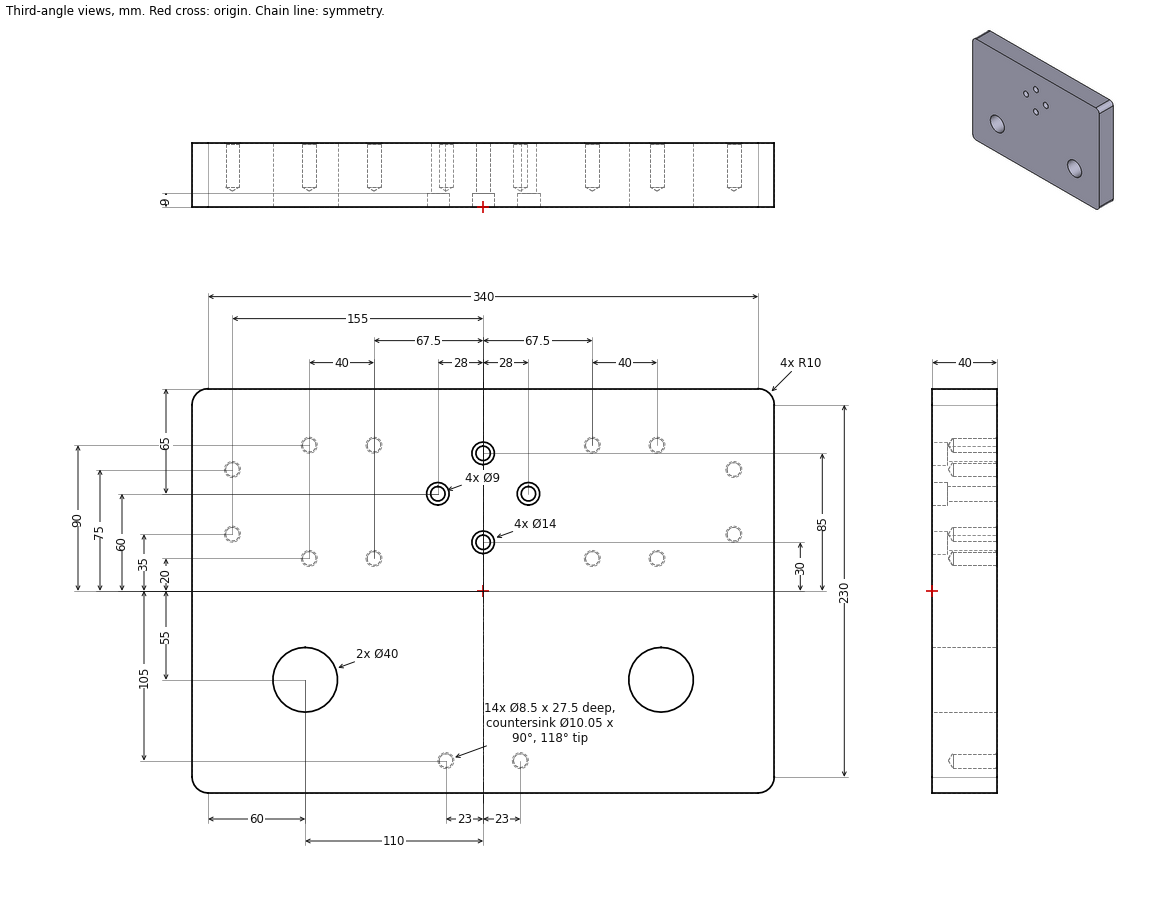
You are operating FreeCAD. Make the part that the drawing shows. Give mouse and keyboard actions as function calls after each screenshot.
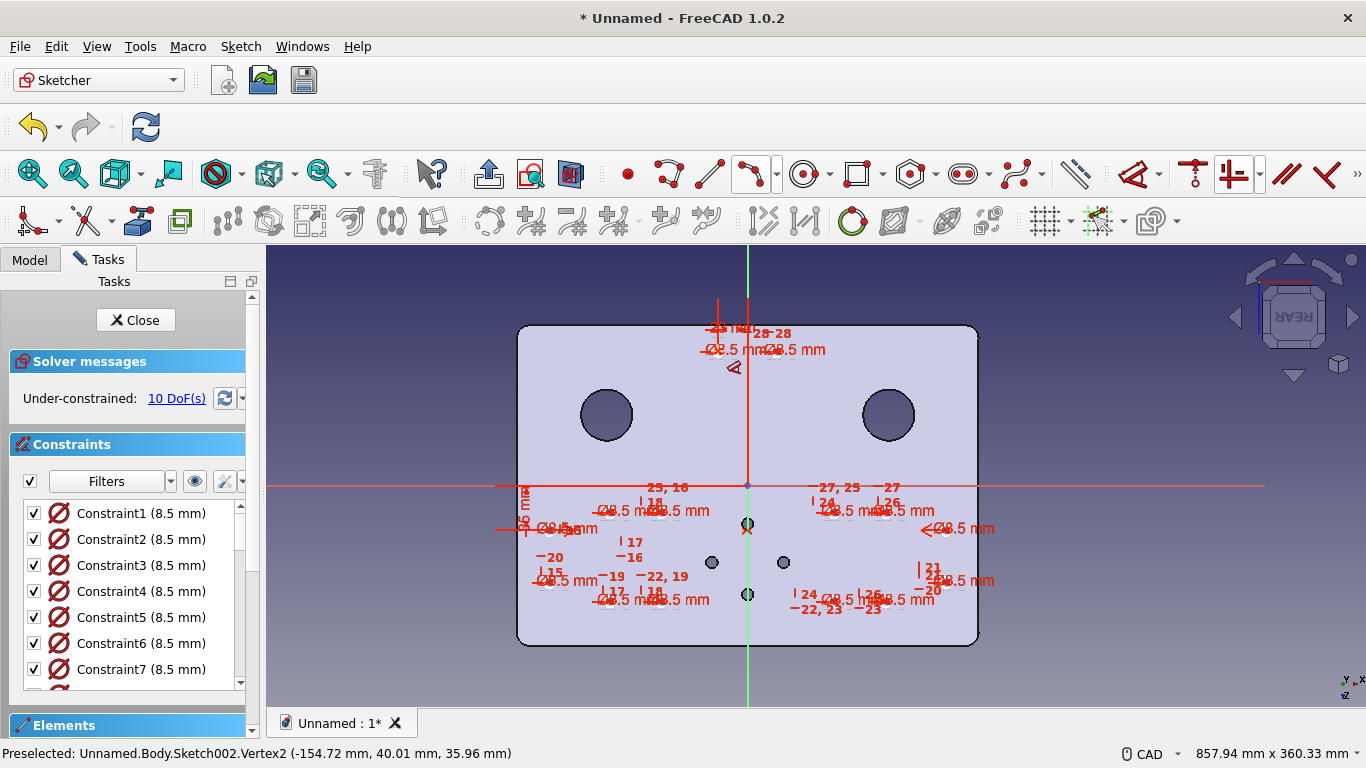
click(549, 583)
click(515, 534)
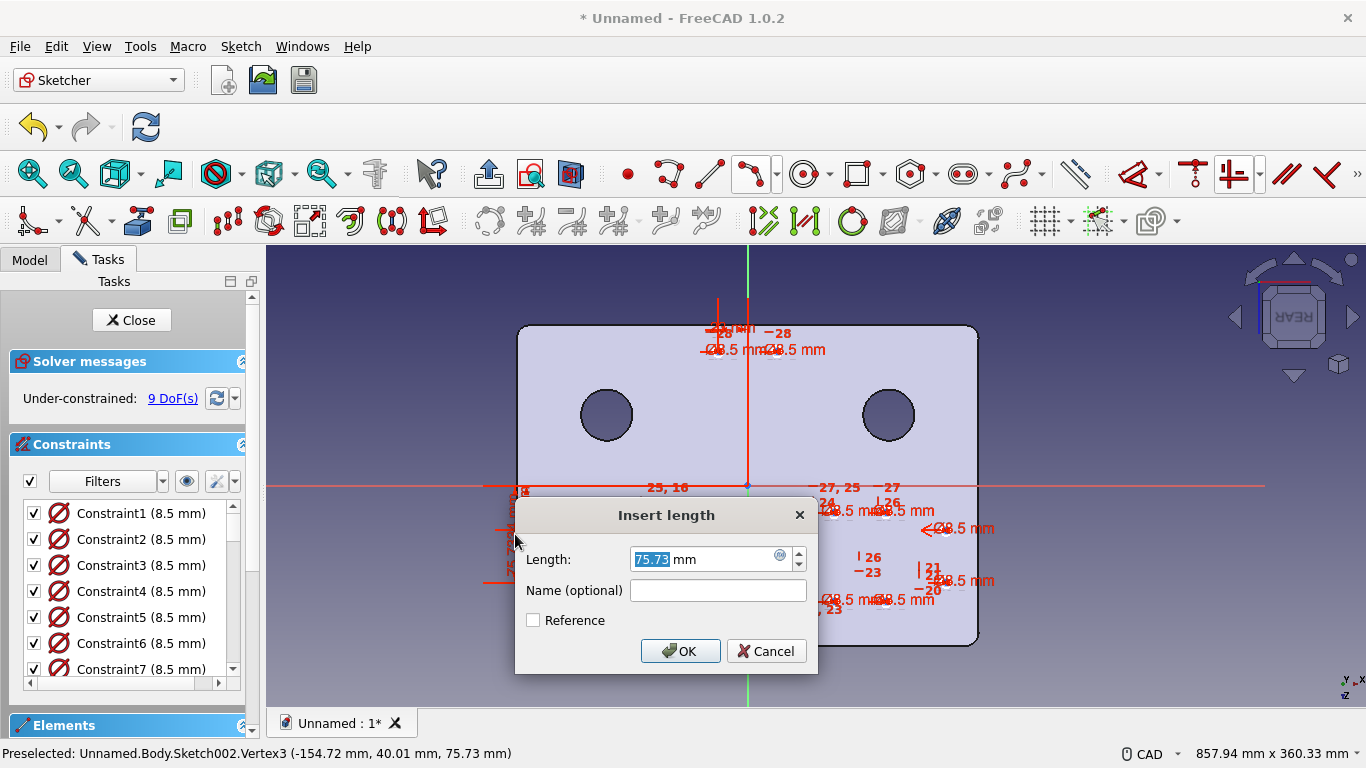
text(75)
key(Return)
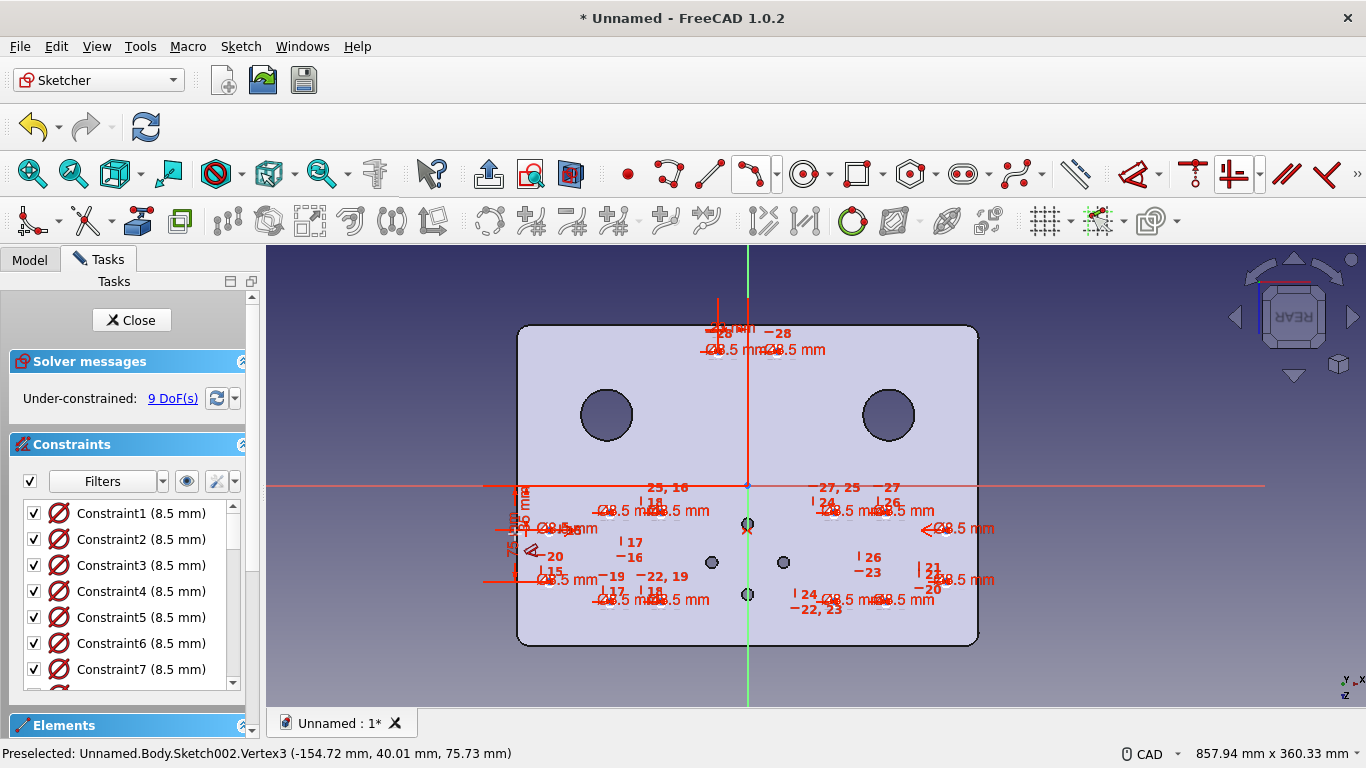
scroll(610, 513, up, 3)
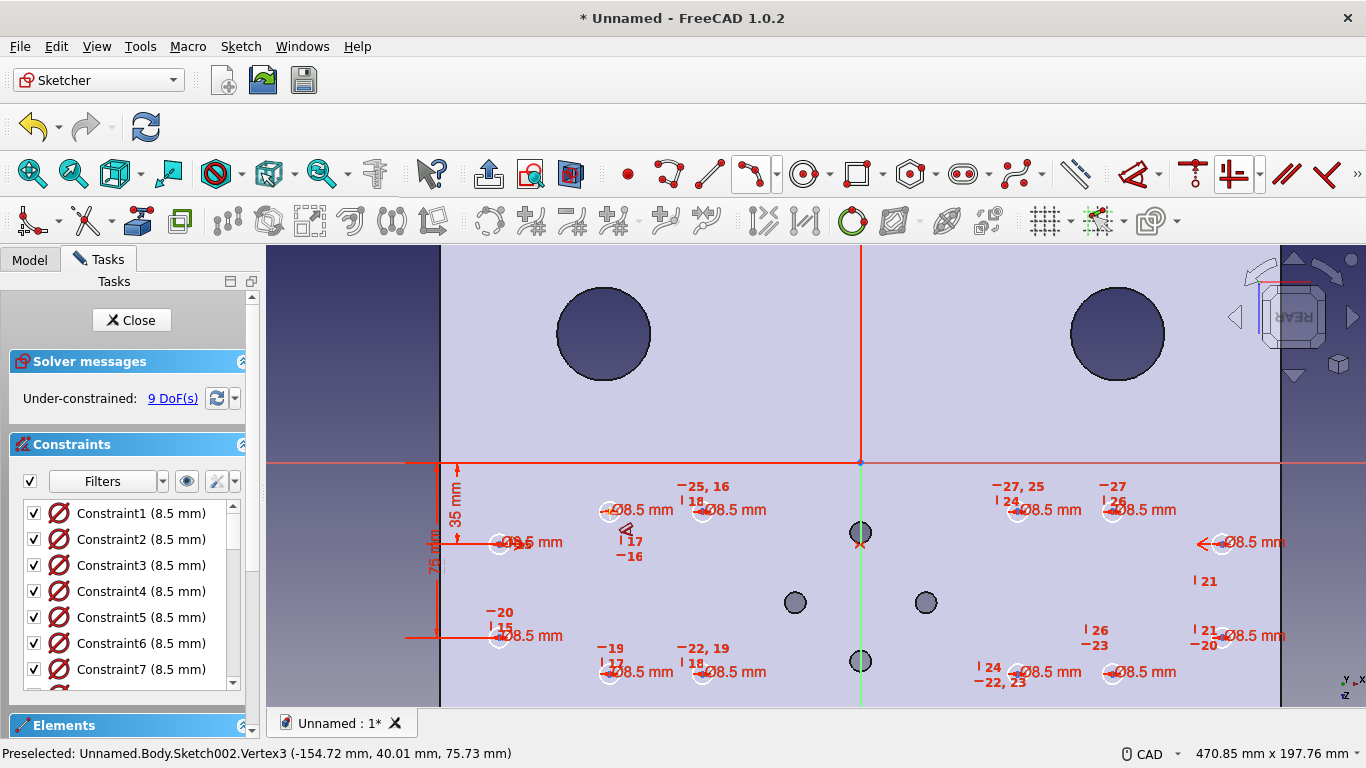
click(610, 512)
click(576, 487)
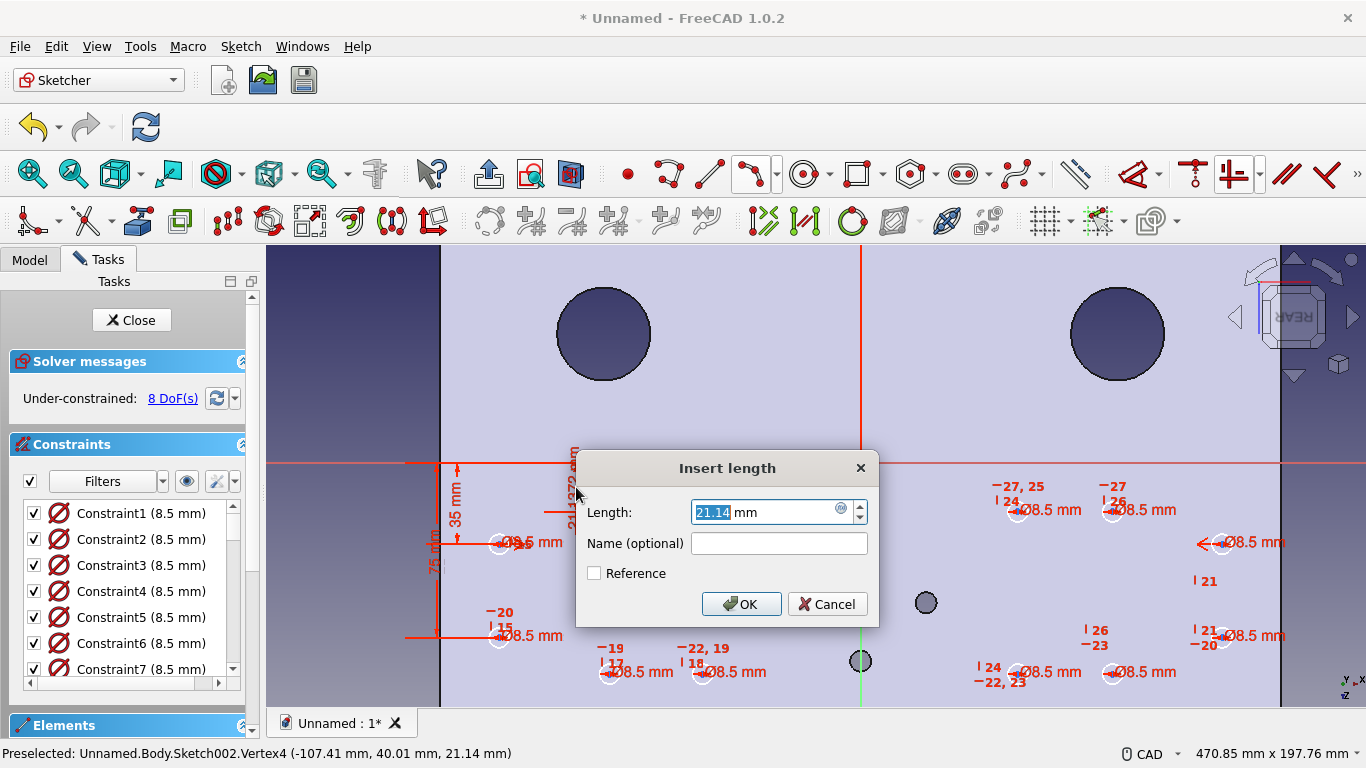
text(20)
key(Return)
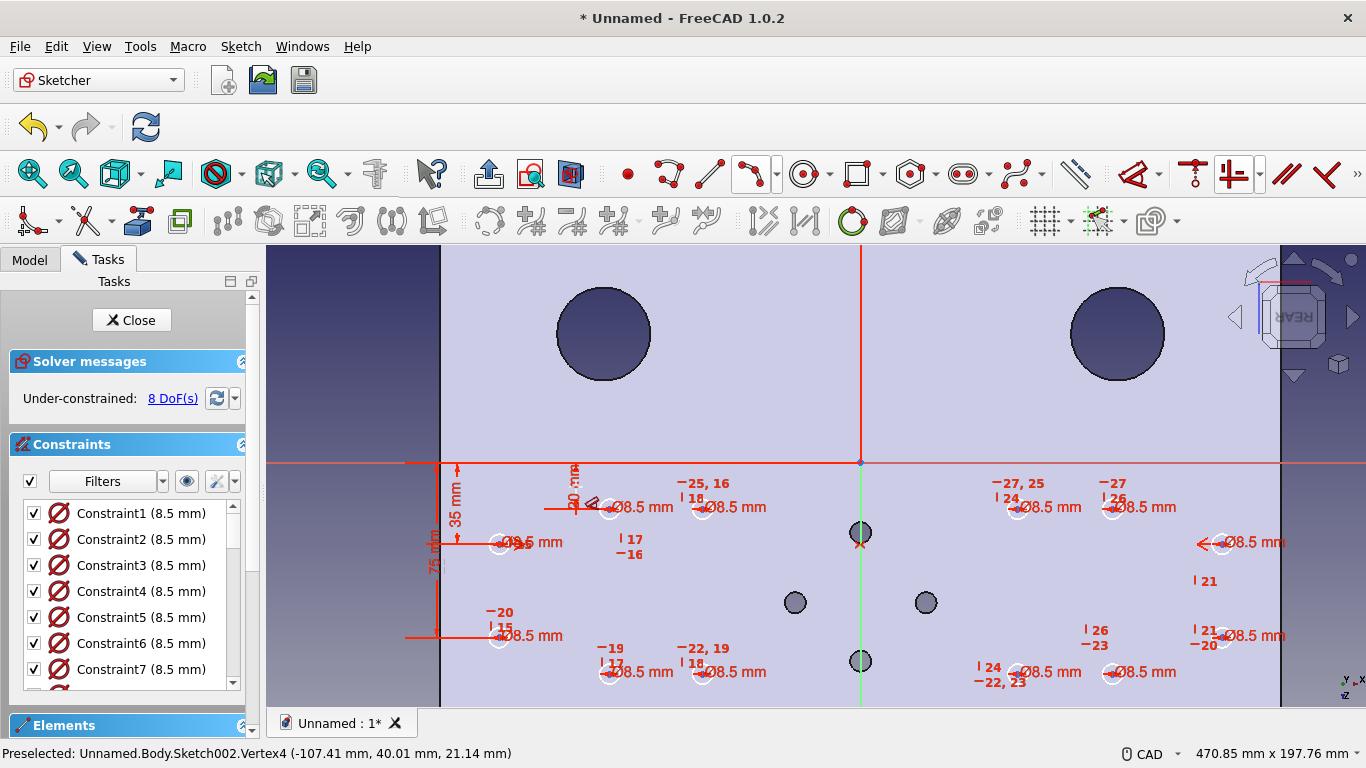
click(610, 674)
click(576, 568)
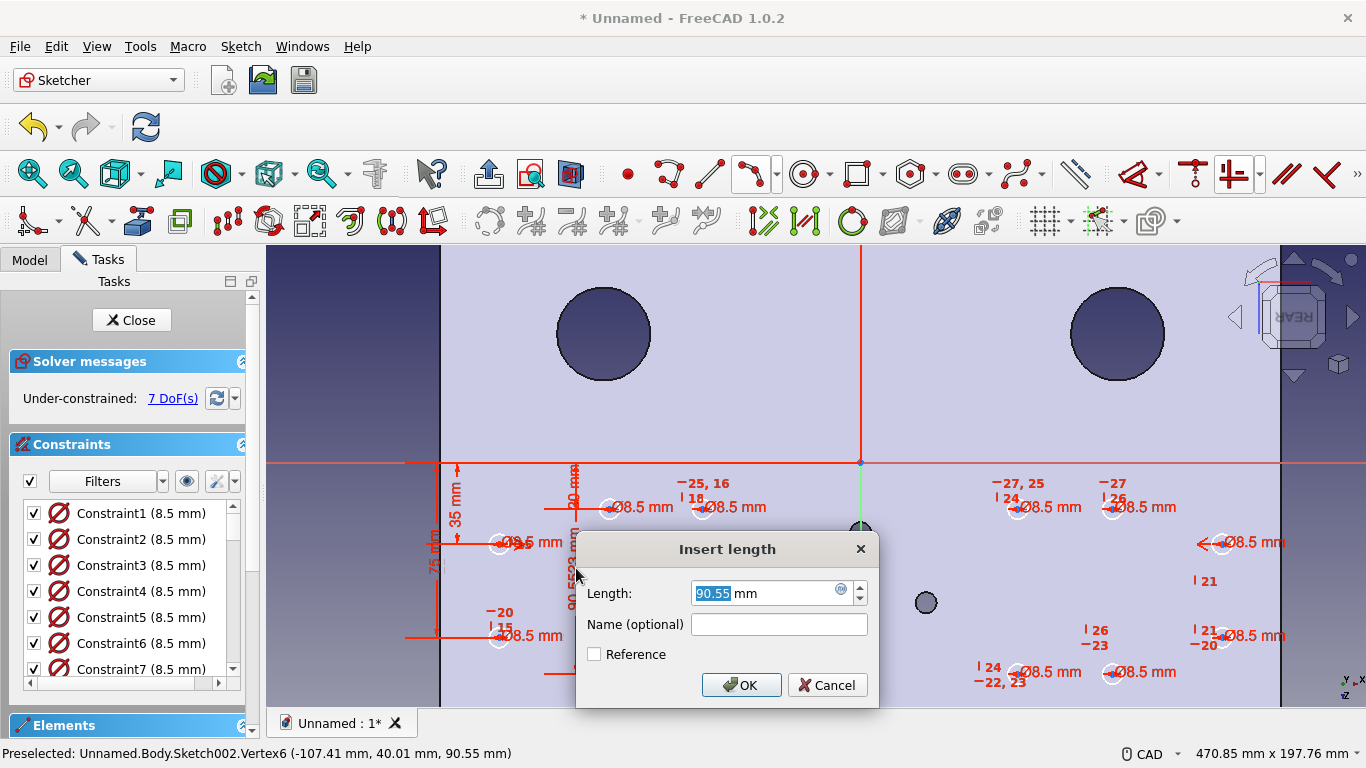
text(90)
key(Return)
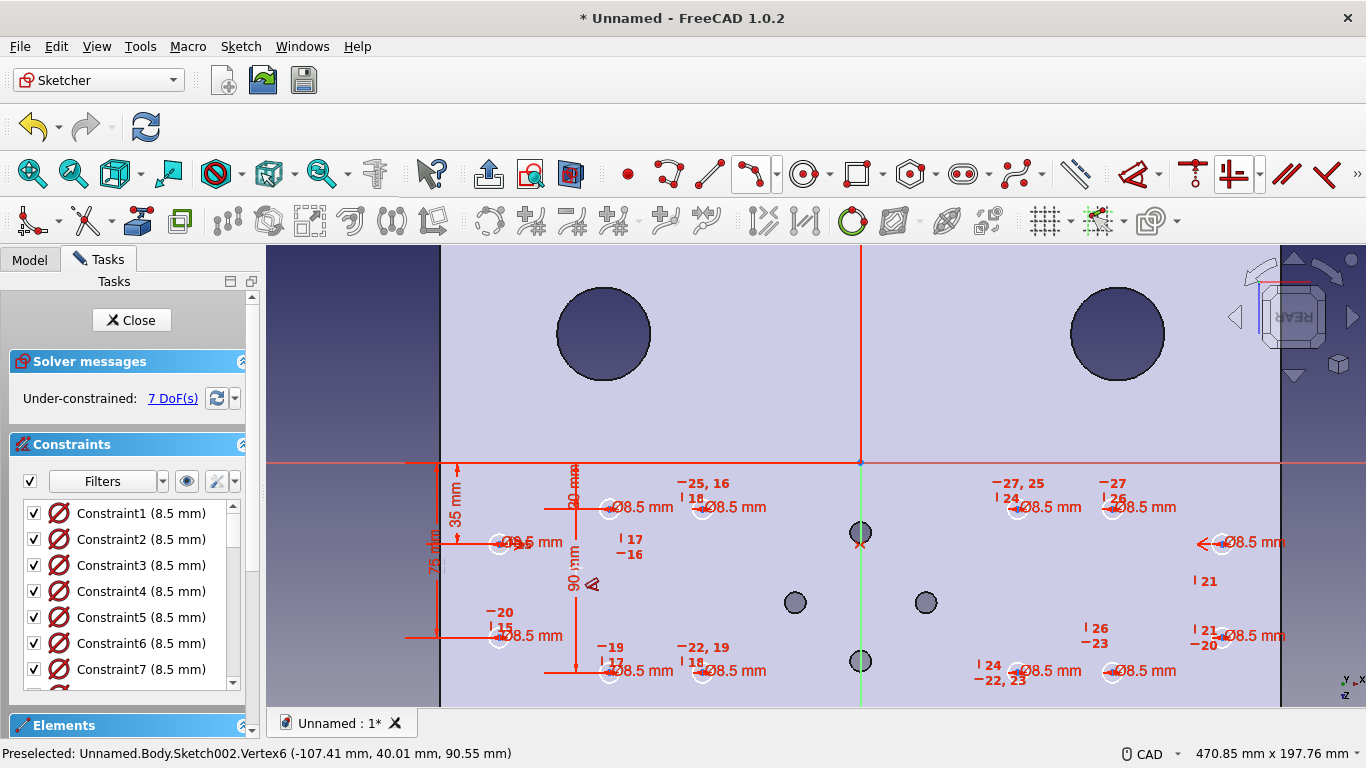
scroll(610, 514, down, 3)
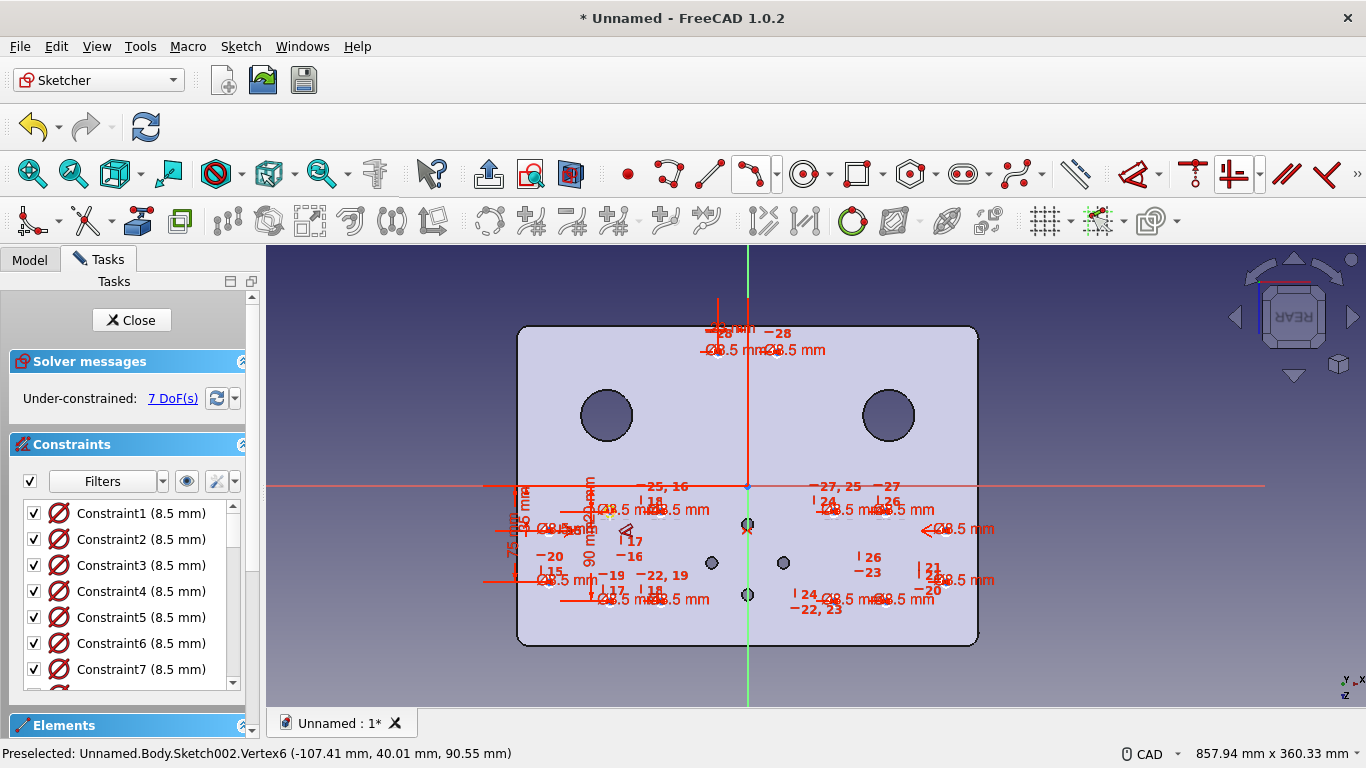
scroll(777, 352, up, 2)